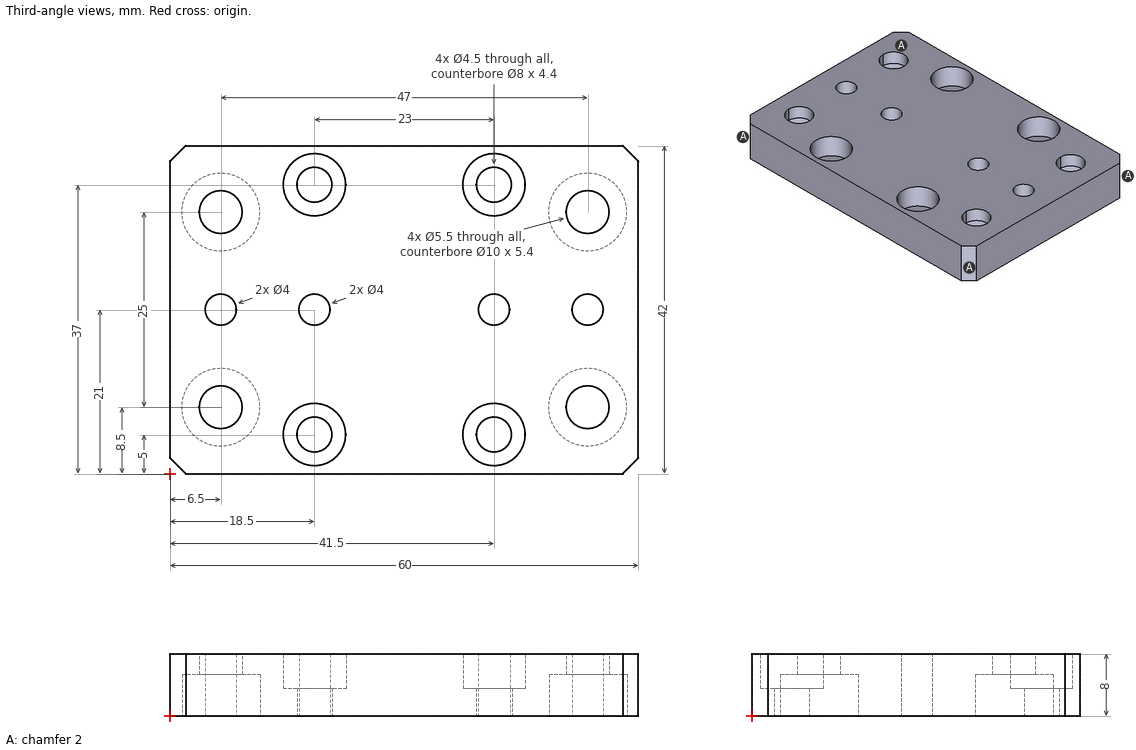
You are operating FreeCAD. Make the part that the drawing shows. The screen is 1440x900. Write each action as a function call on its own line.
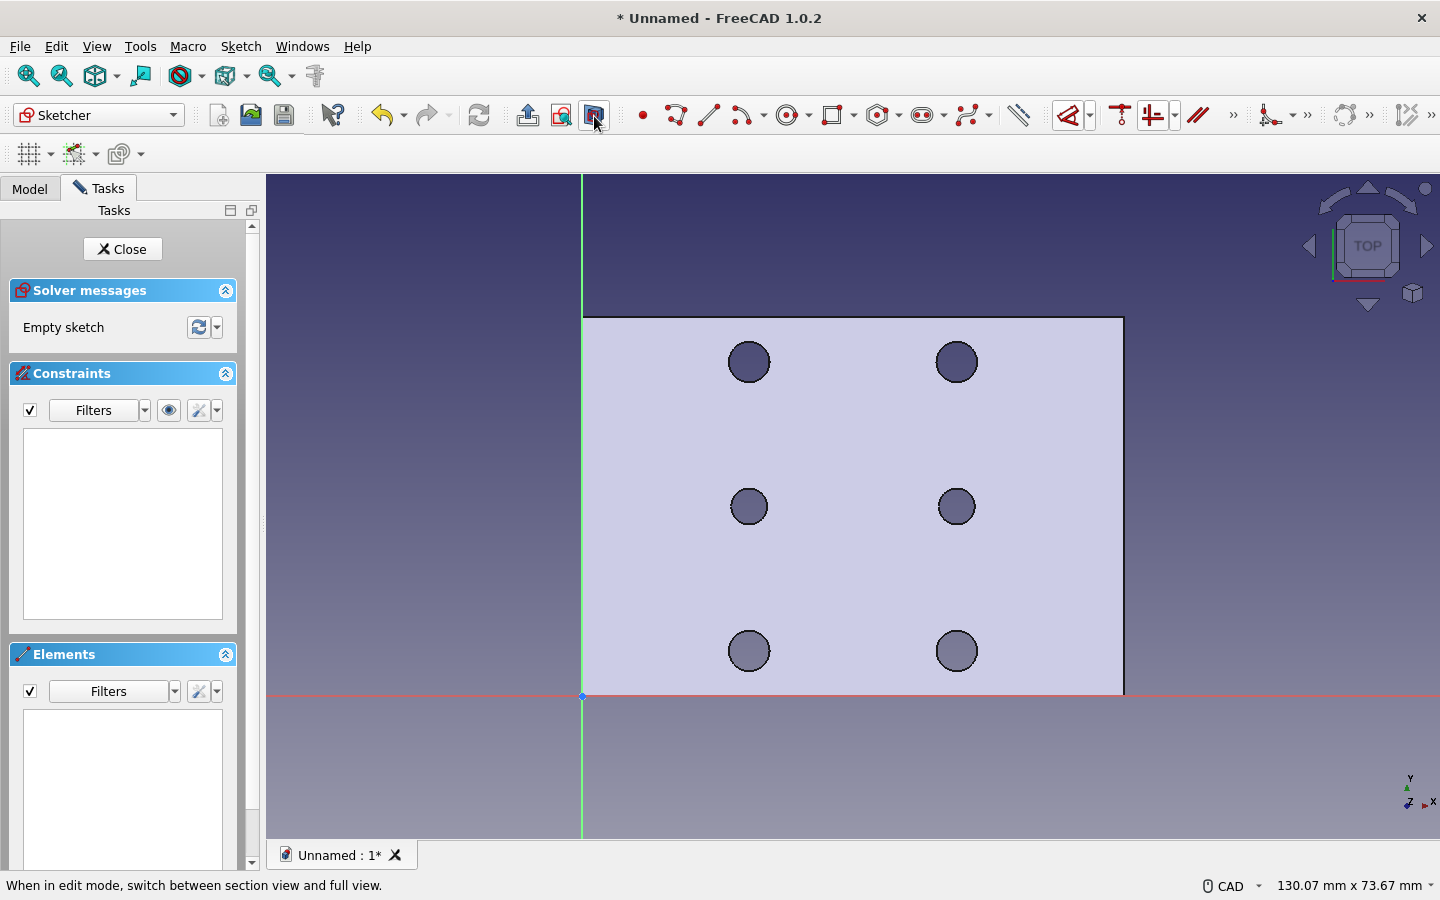
click(786, 116)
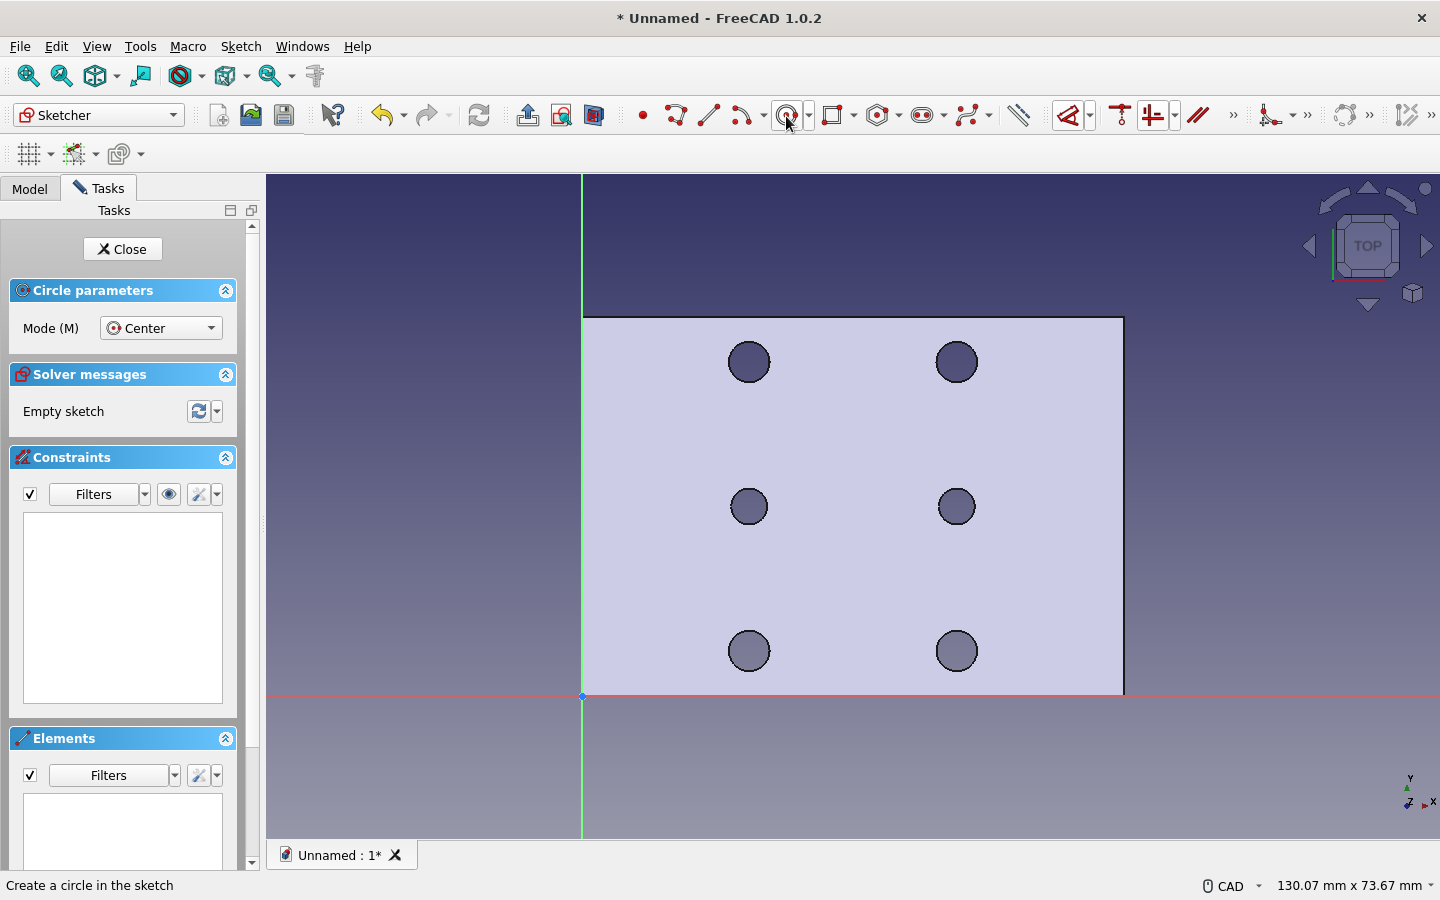
click(1065, 394)
click(1083, 376)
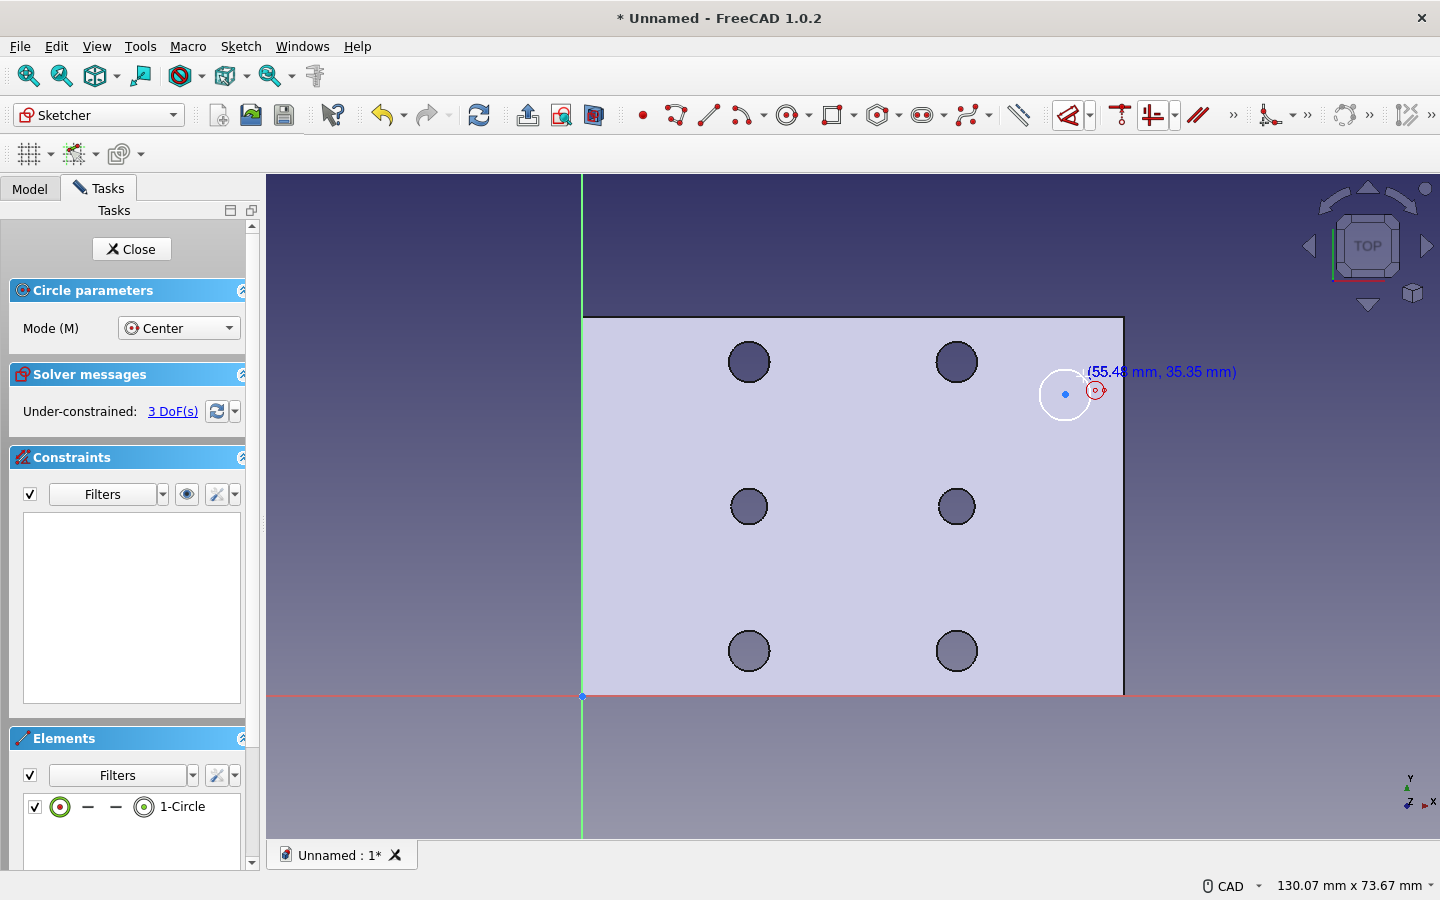
click(641, 394)
click(658, 376)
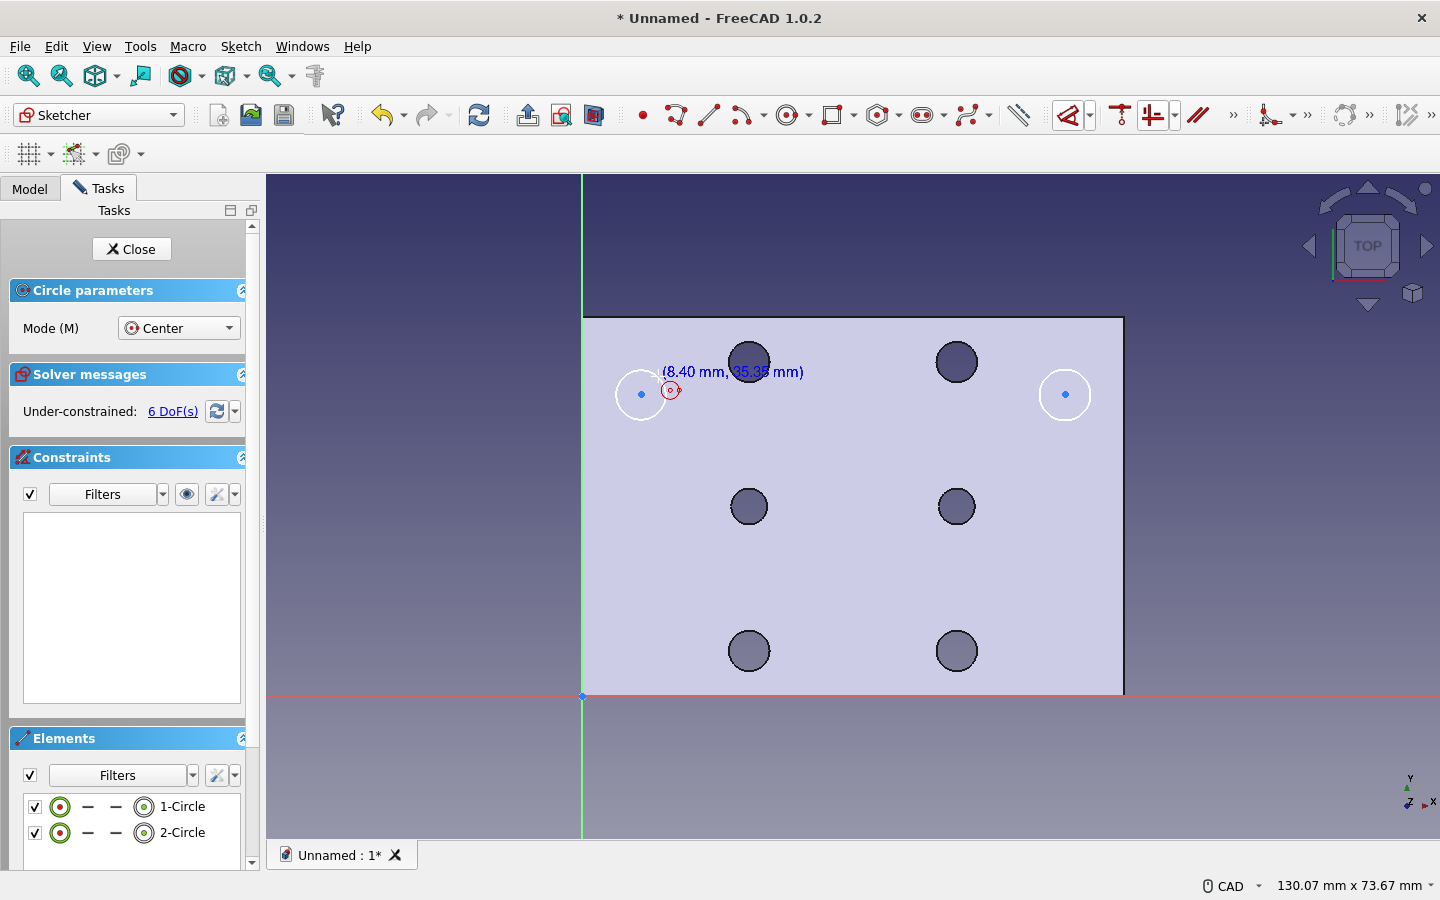
click(641, 619)
click(658, 602)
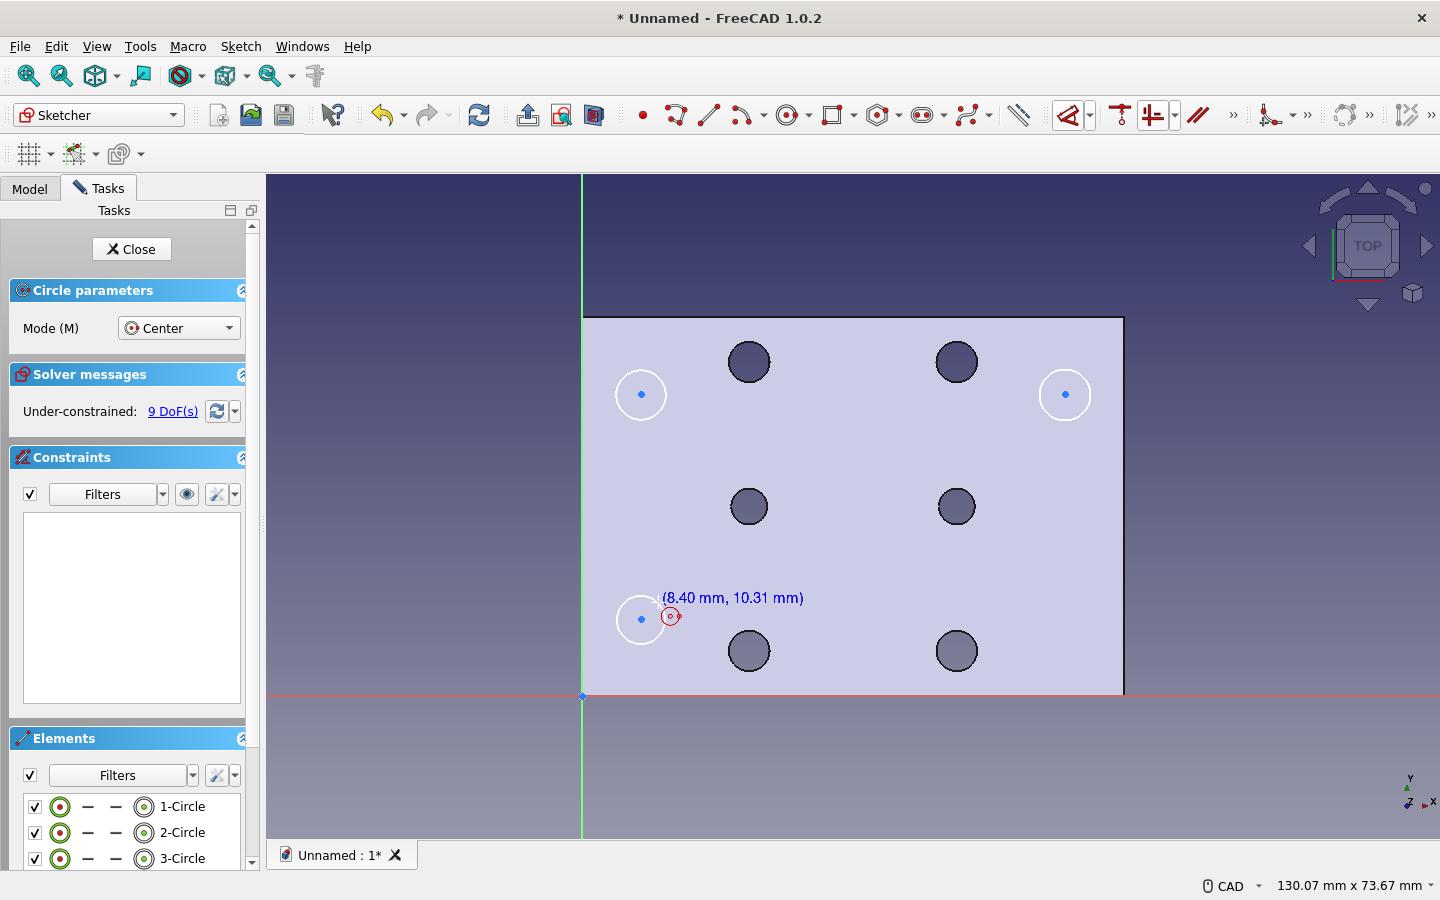
click(1065, 619)
click(1083, 602)
key(Escape)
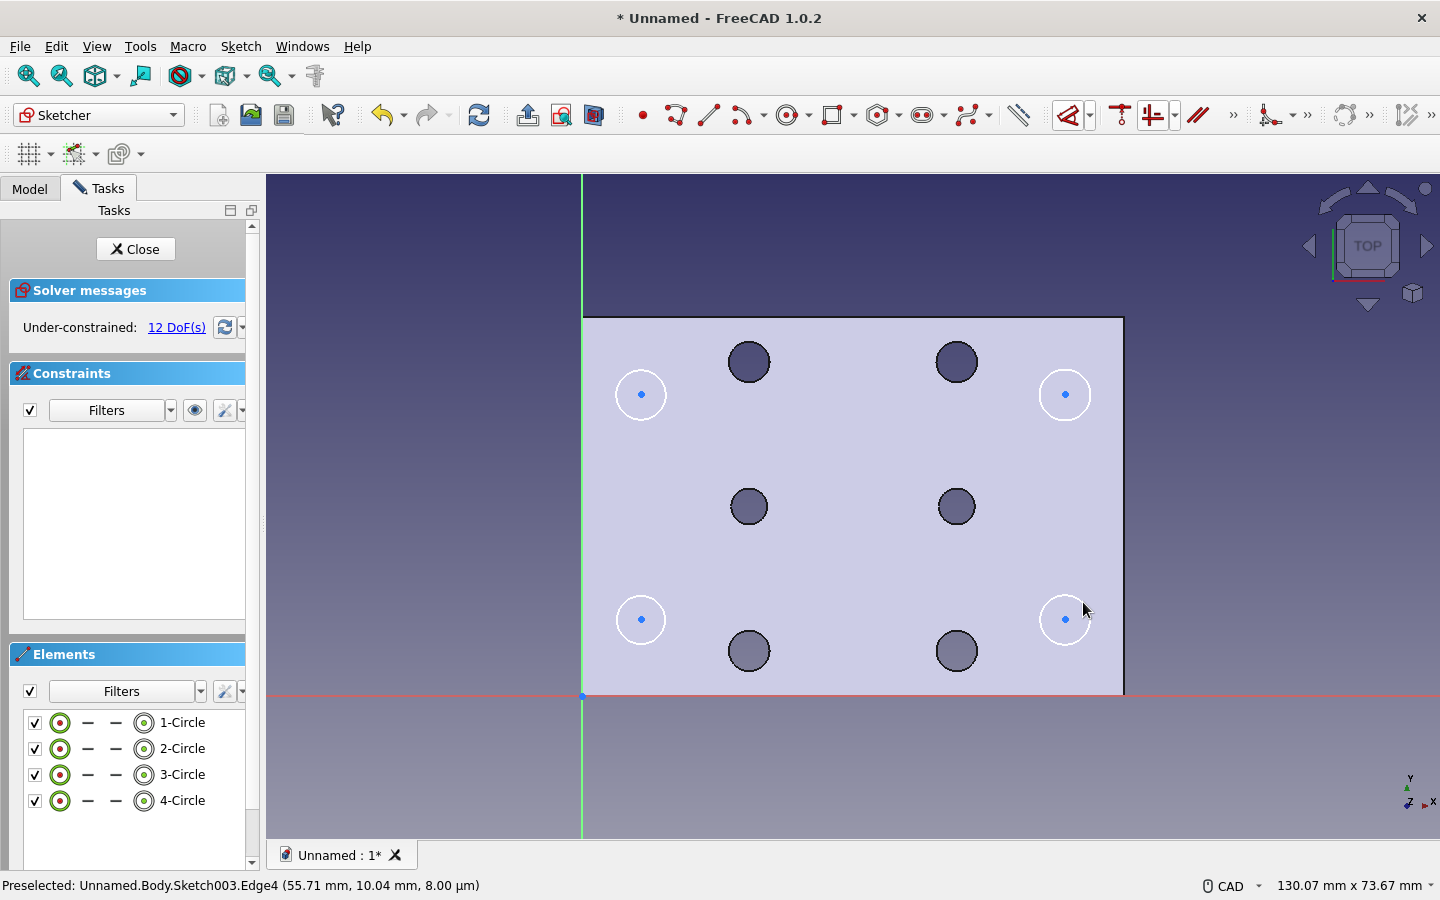
click(1083, 377)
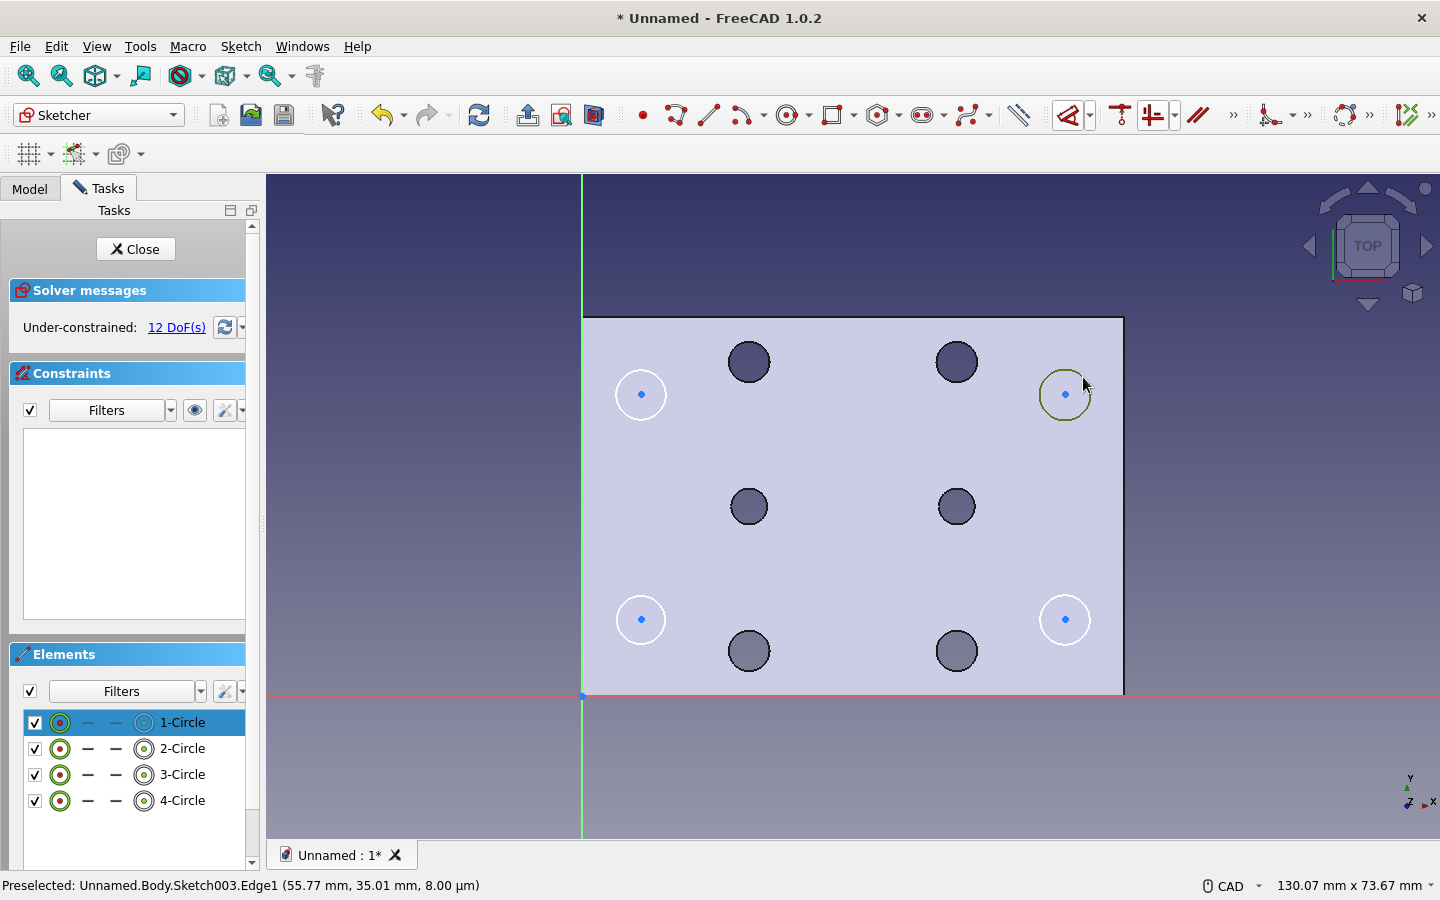
click(658, 377)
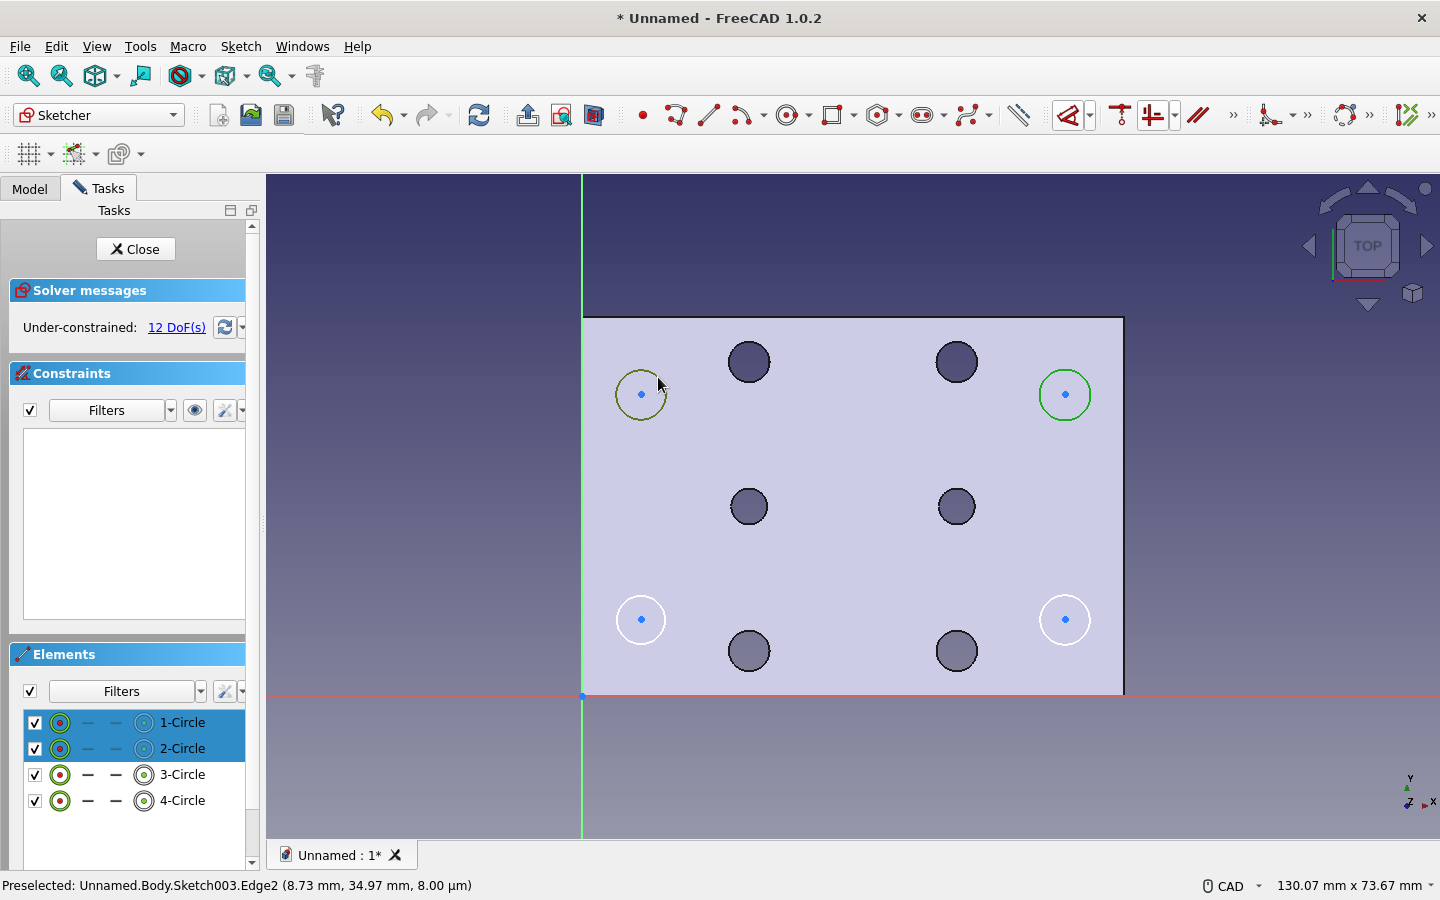
click(658, 603)